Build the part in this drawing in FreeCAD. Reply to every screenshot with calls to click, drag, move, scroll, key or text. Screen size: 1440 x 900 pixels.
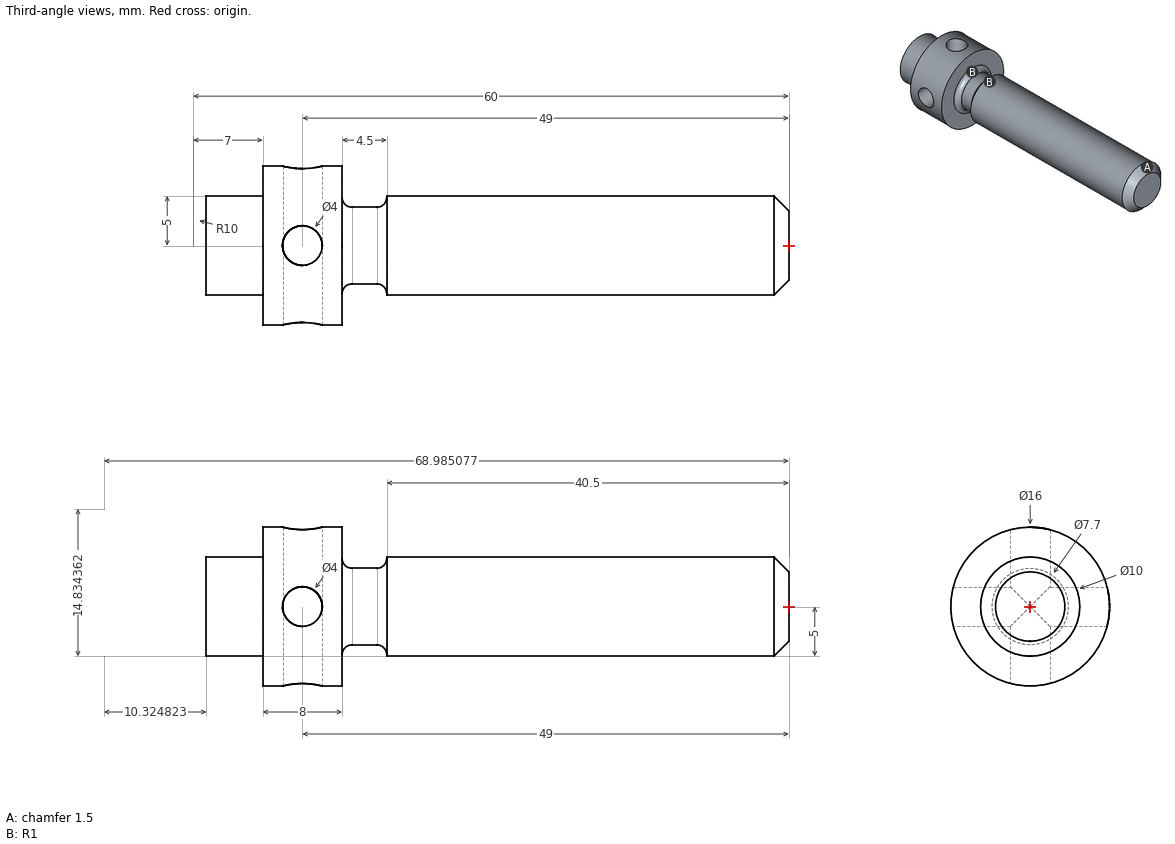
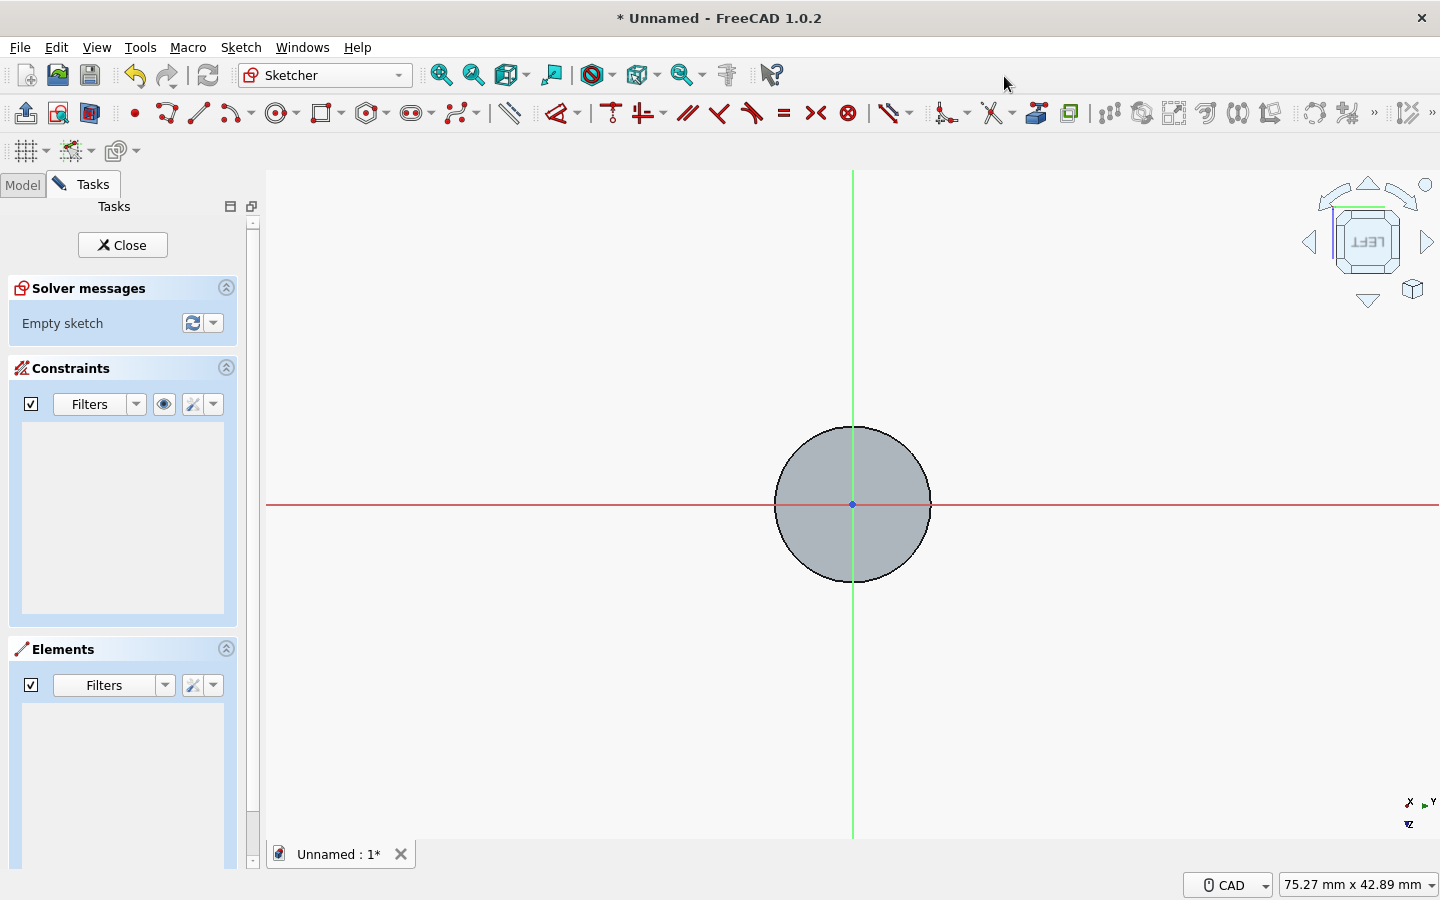
scroll(882, 504, up, 6)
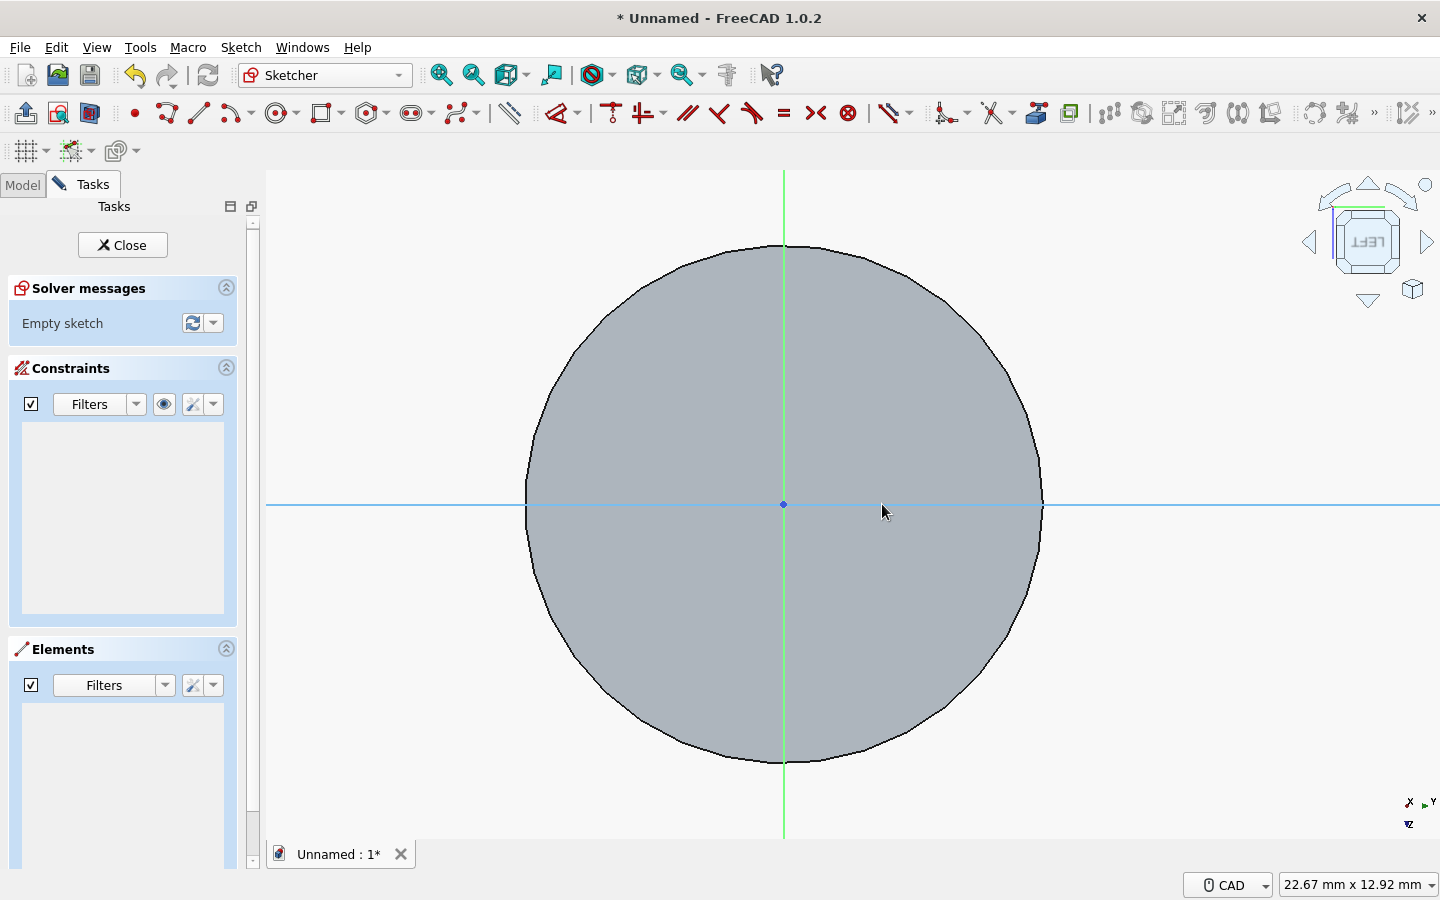
click(276, 114)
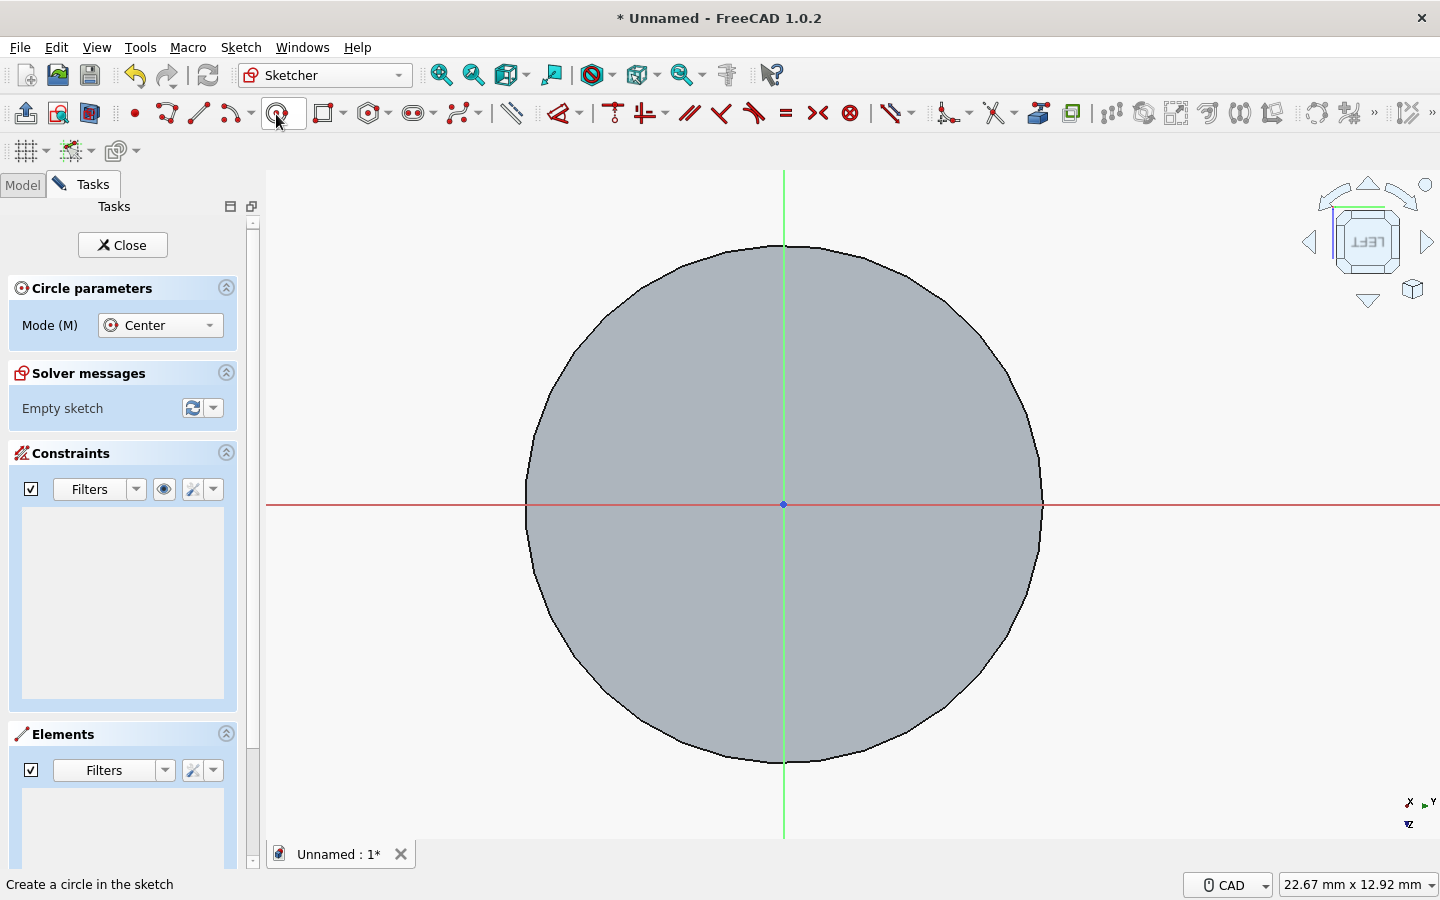
click(784, 504)
click(925, 364)
key(Escape)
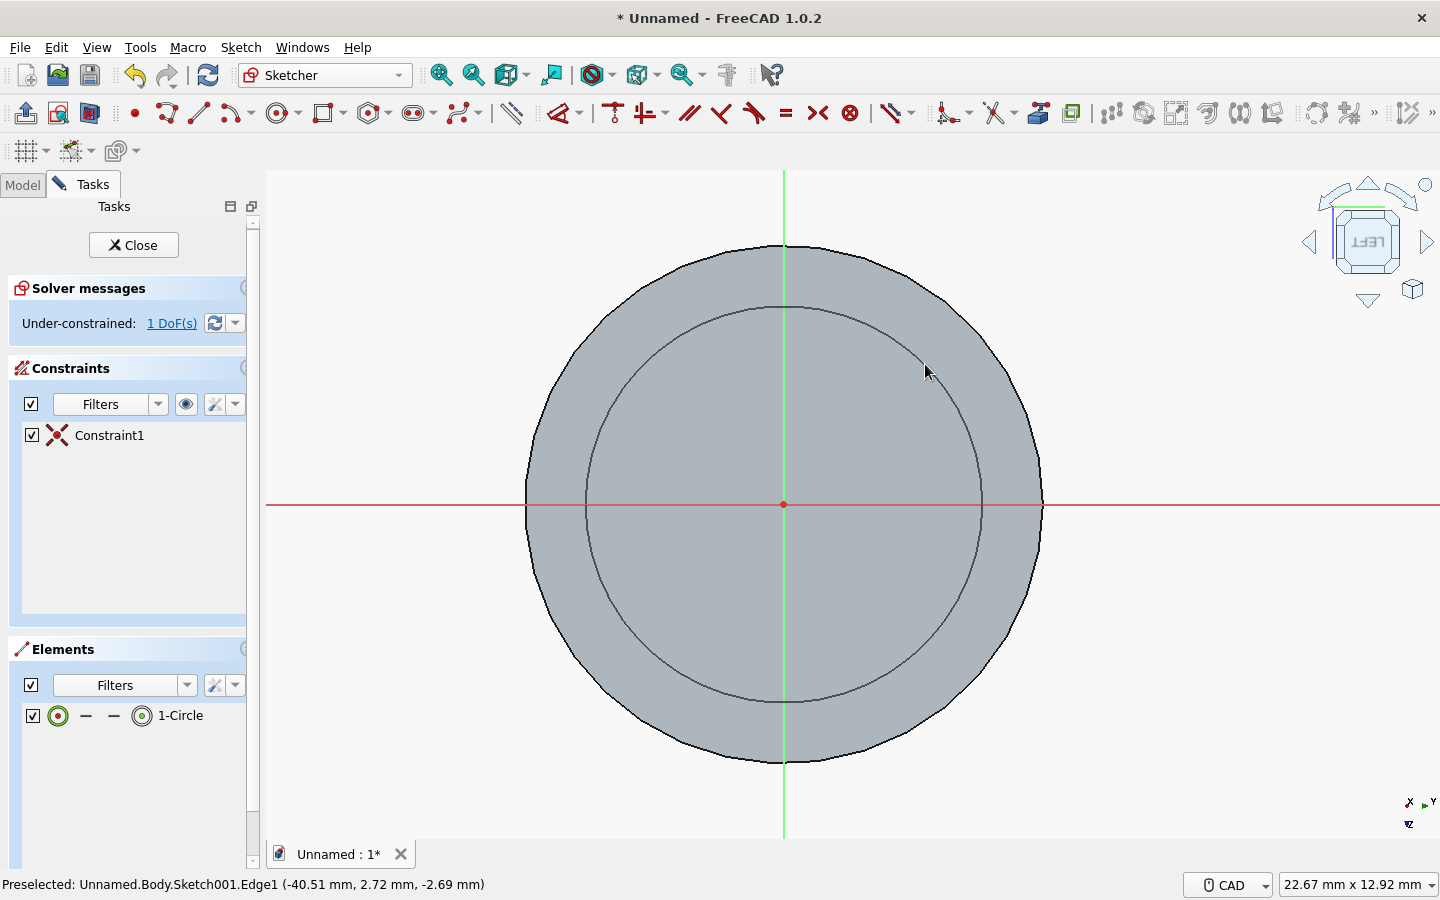
key(d)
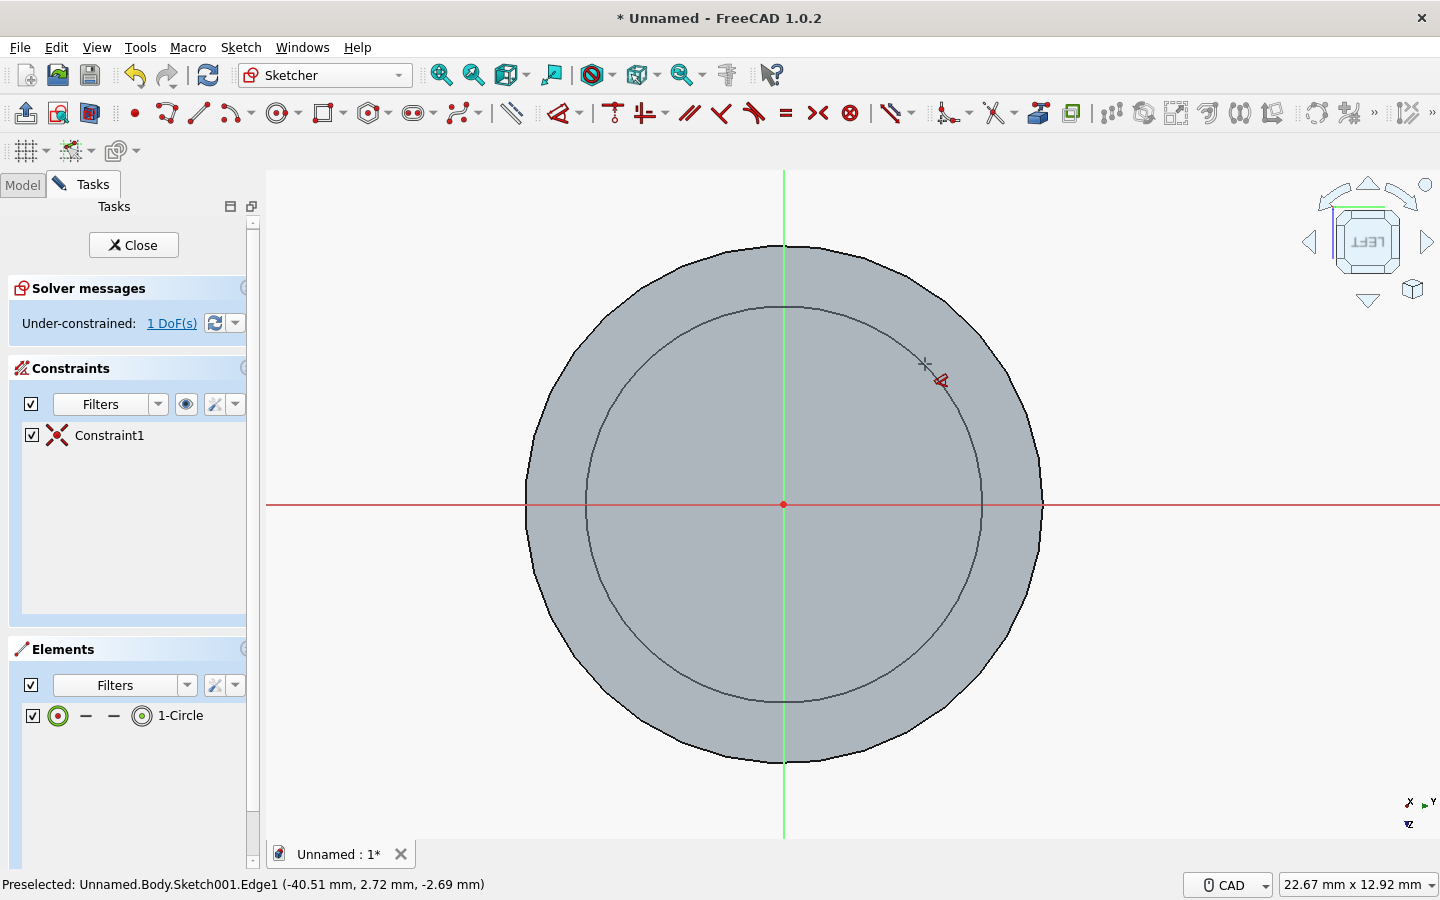
click(924, 364)
click(947, 341)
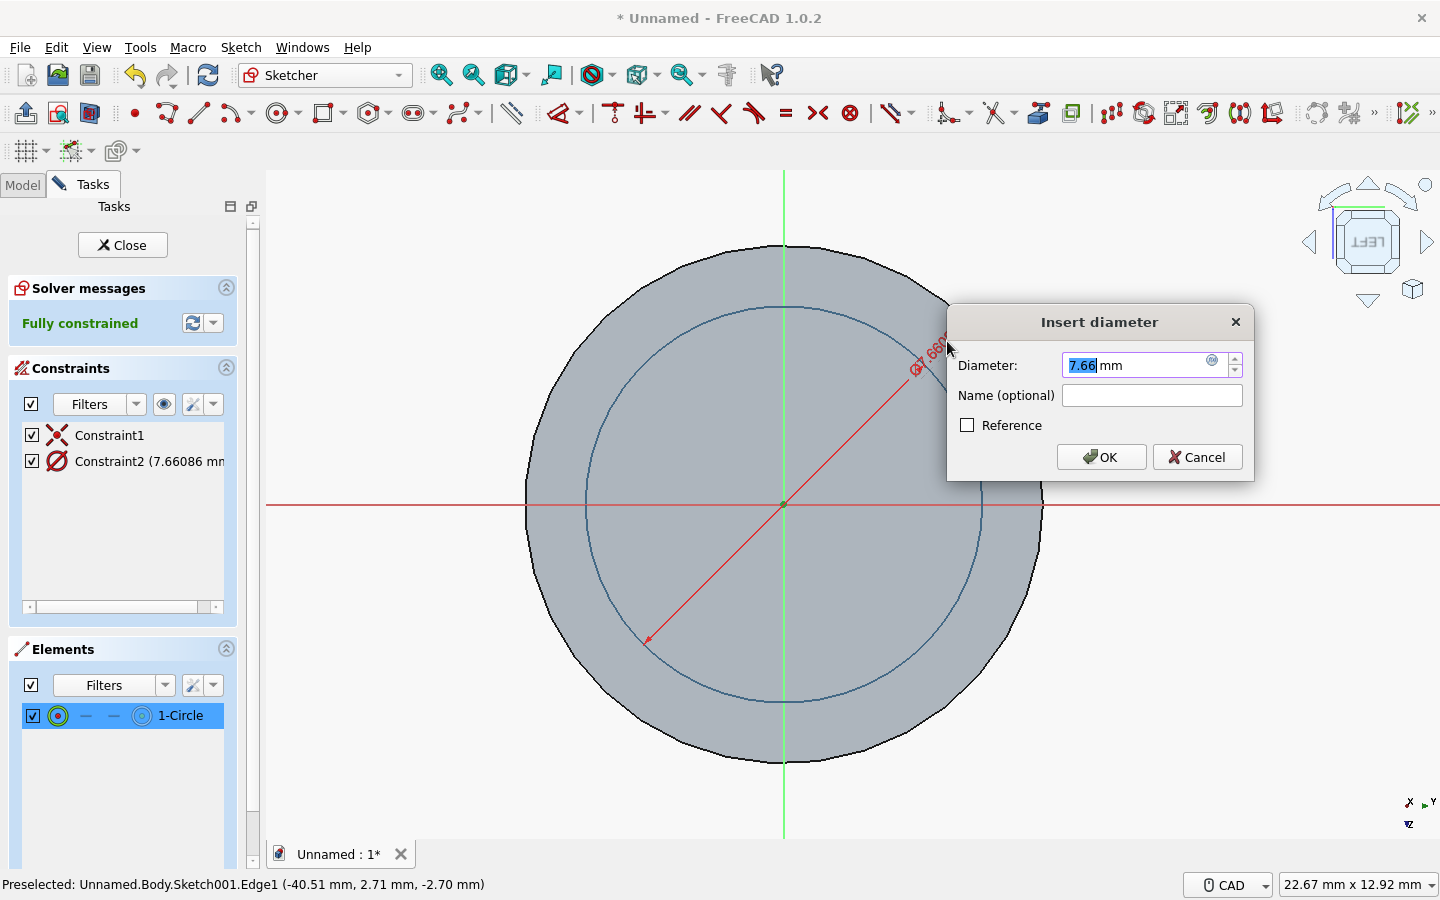
text(7.7)
key(Return)
key(Escape)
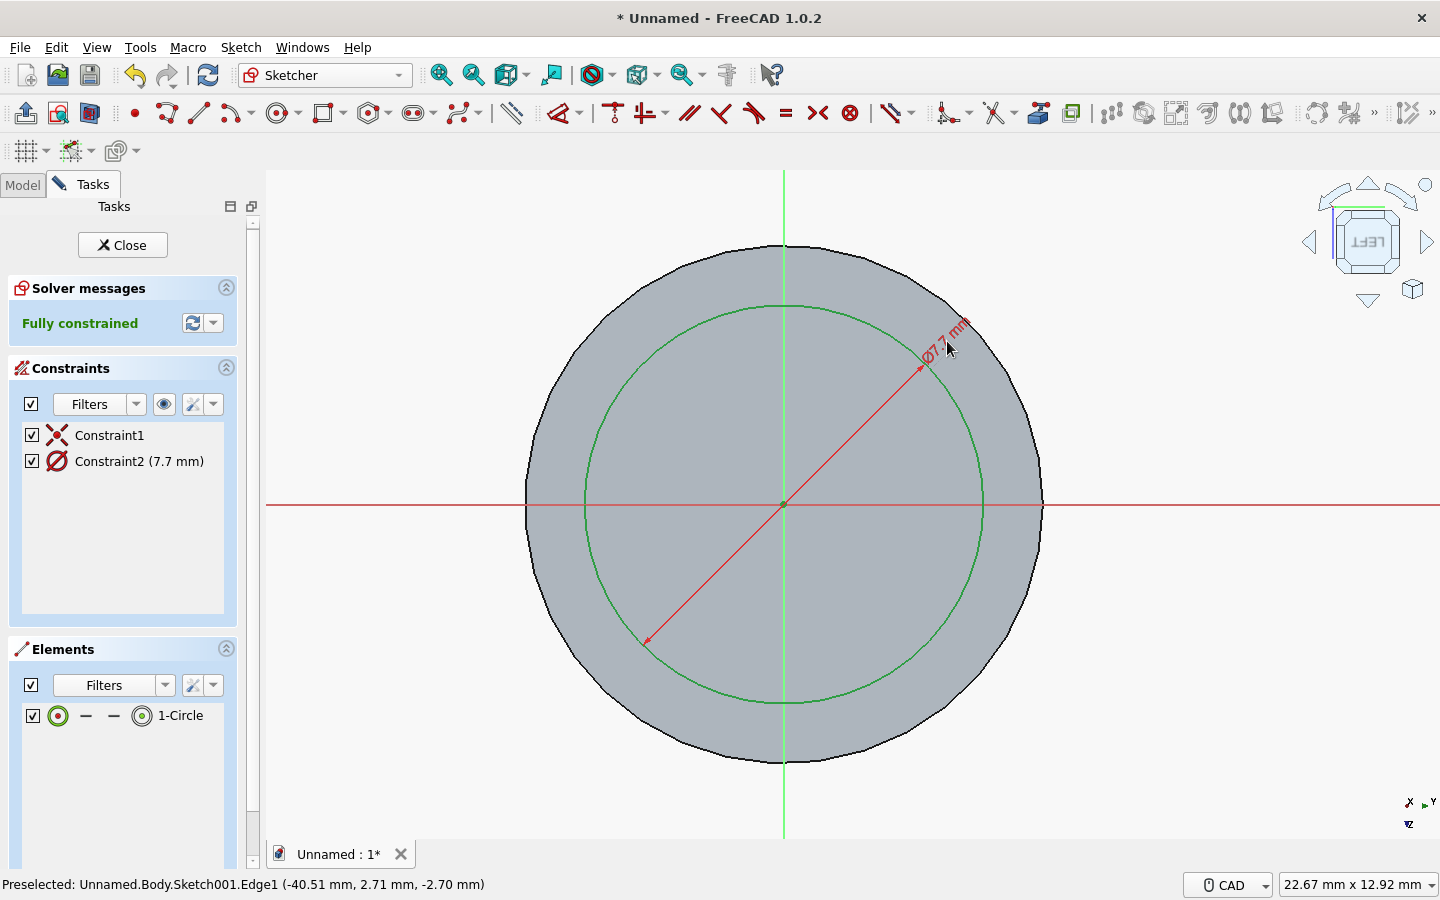
click(123, 245)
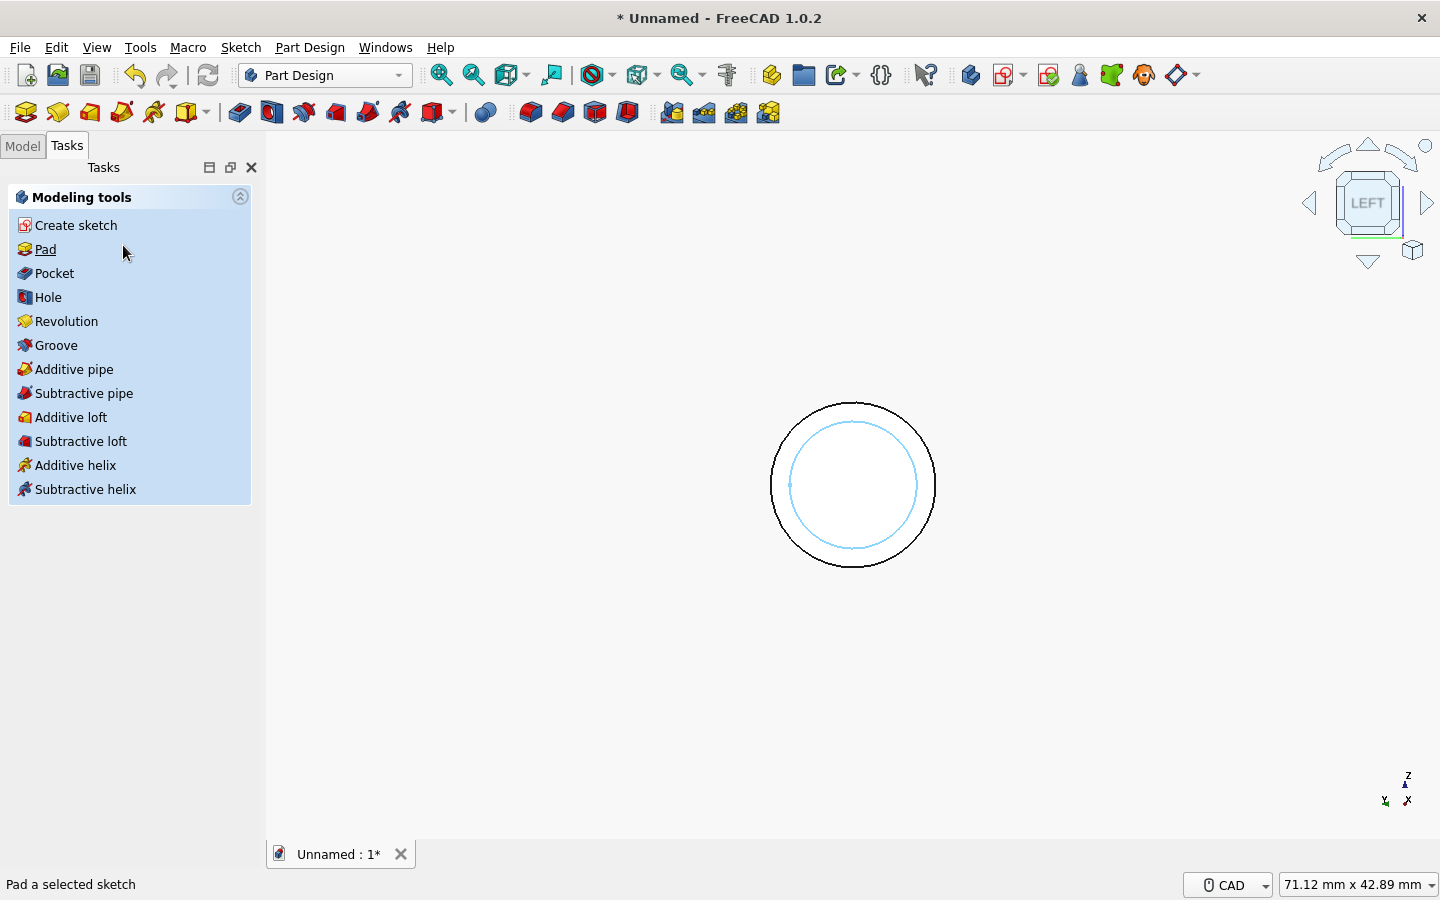
click(26, 112)